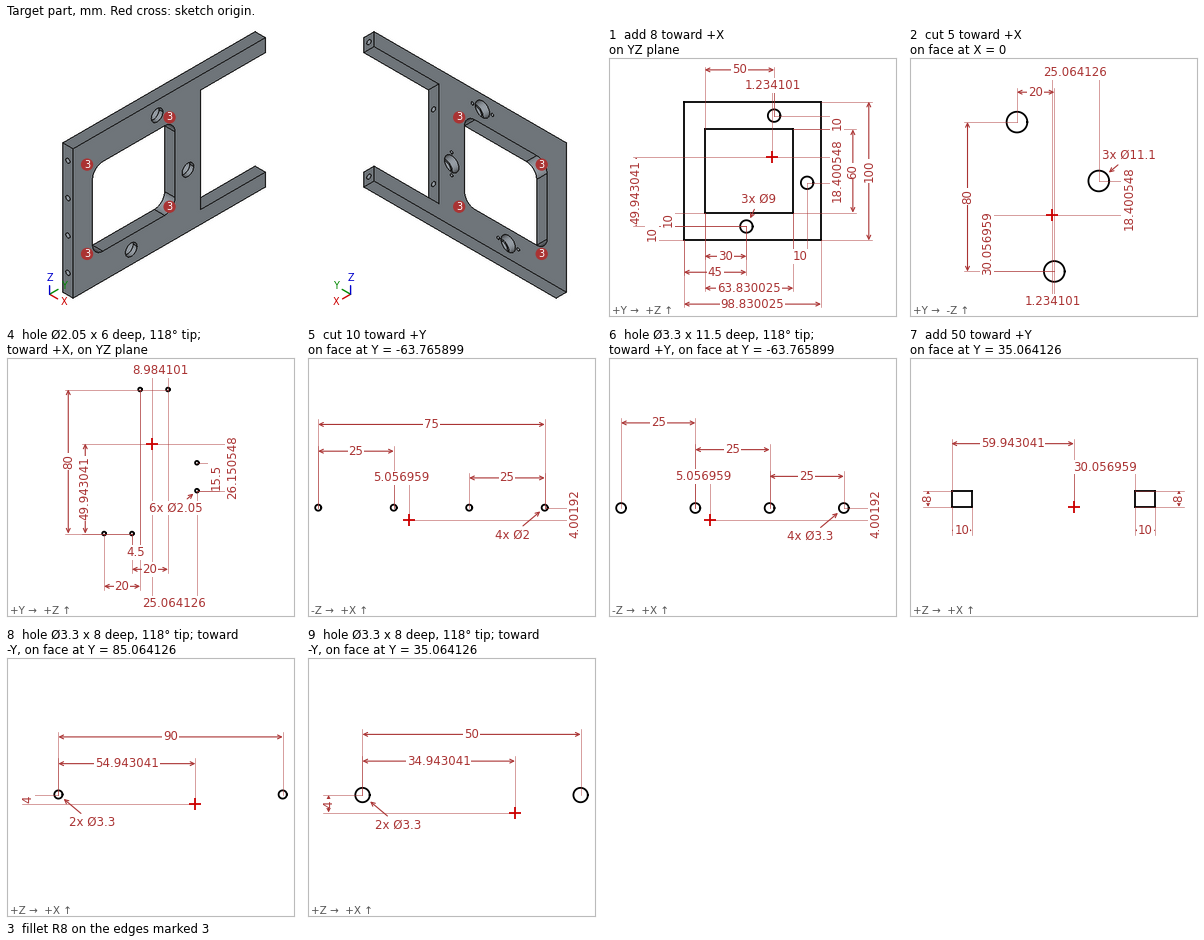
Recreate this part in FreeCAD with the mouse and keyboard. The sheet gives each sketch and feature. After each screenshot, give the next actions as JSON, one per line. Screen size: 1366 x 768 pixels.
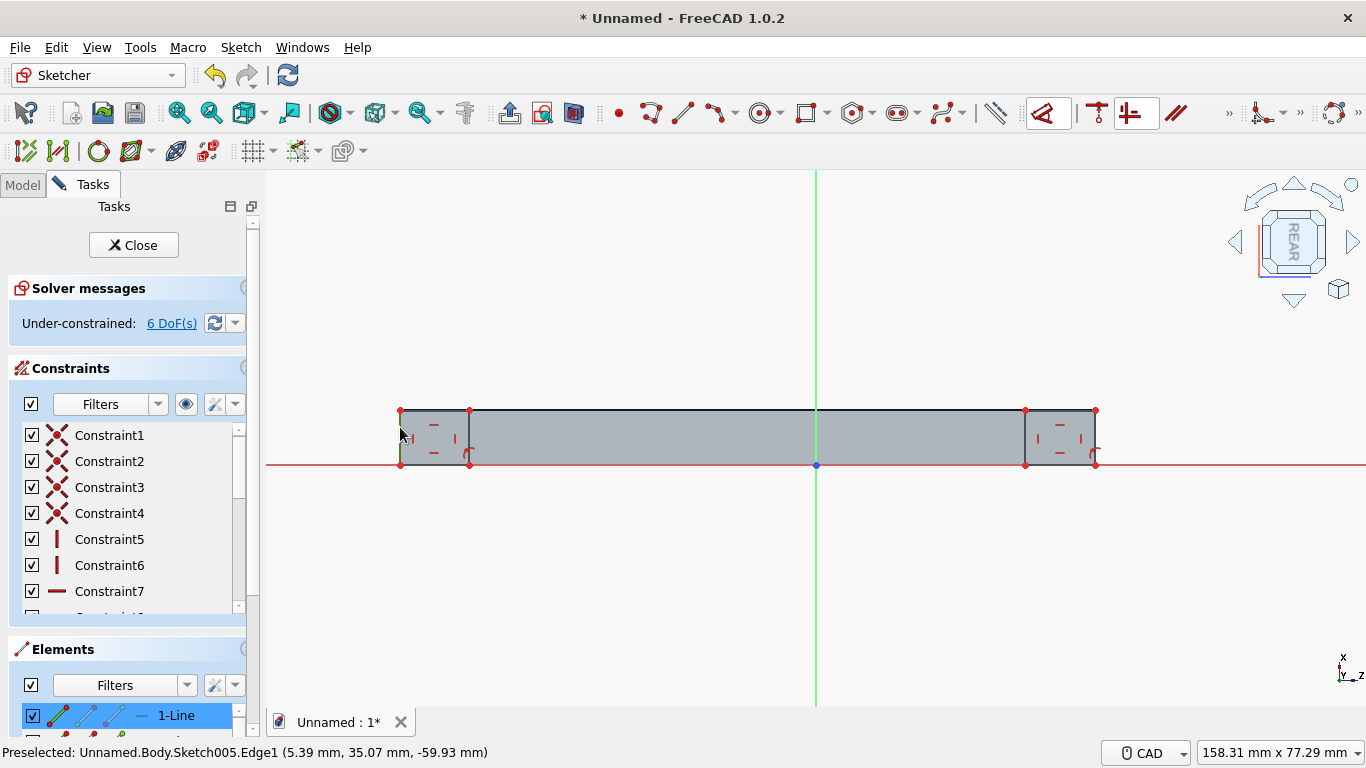
{"action": "left_click", "coordinate": [1066, 114]}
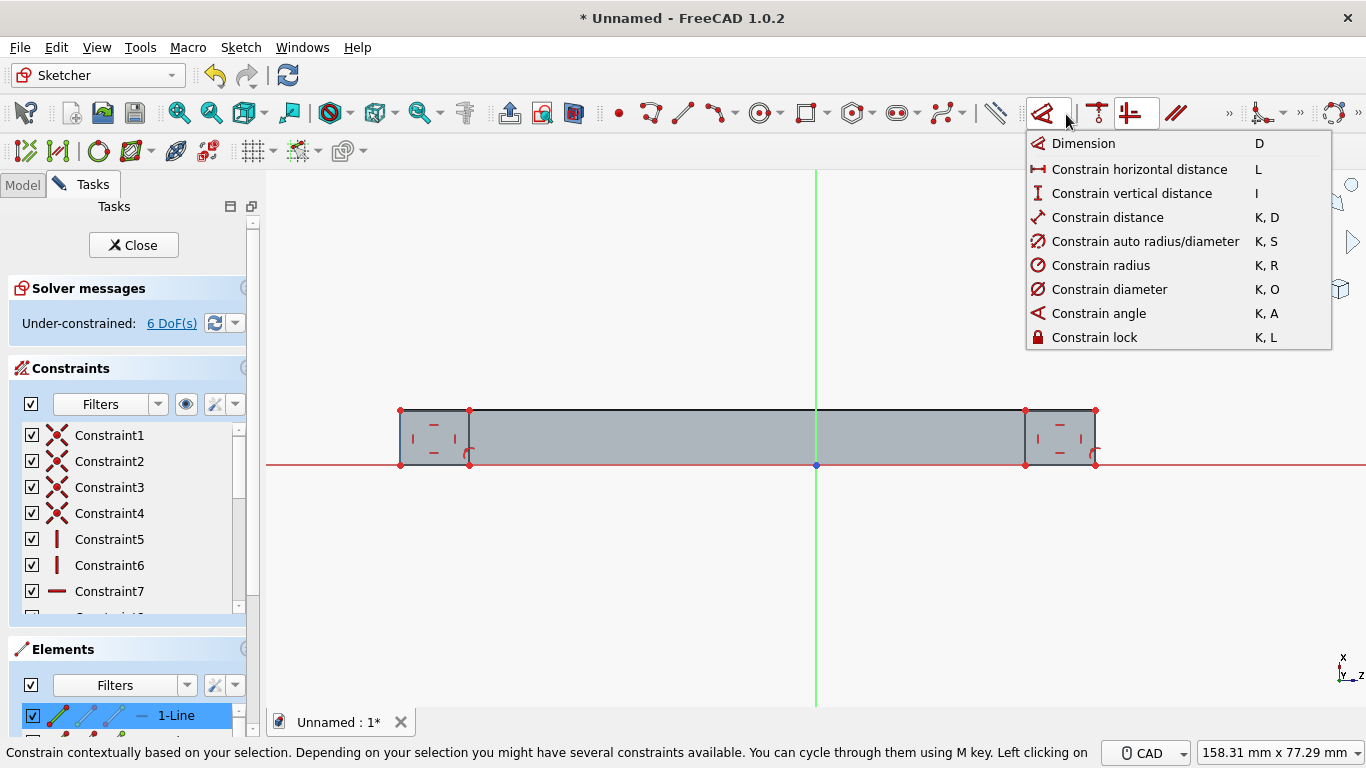
{"action": "left_click", "coordinate": [1179, 193]}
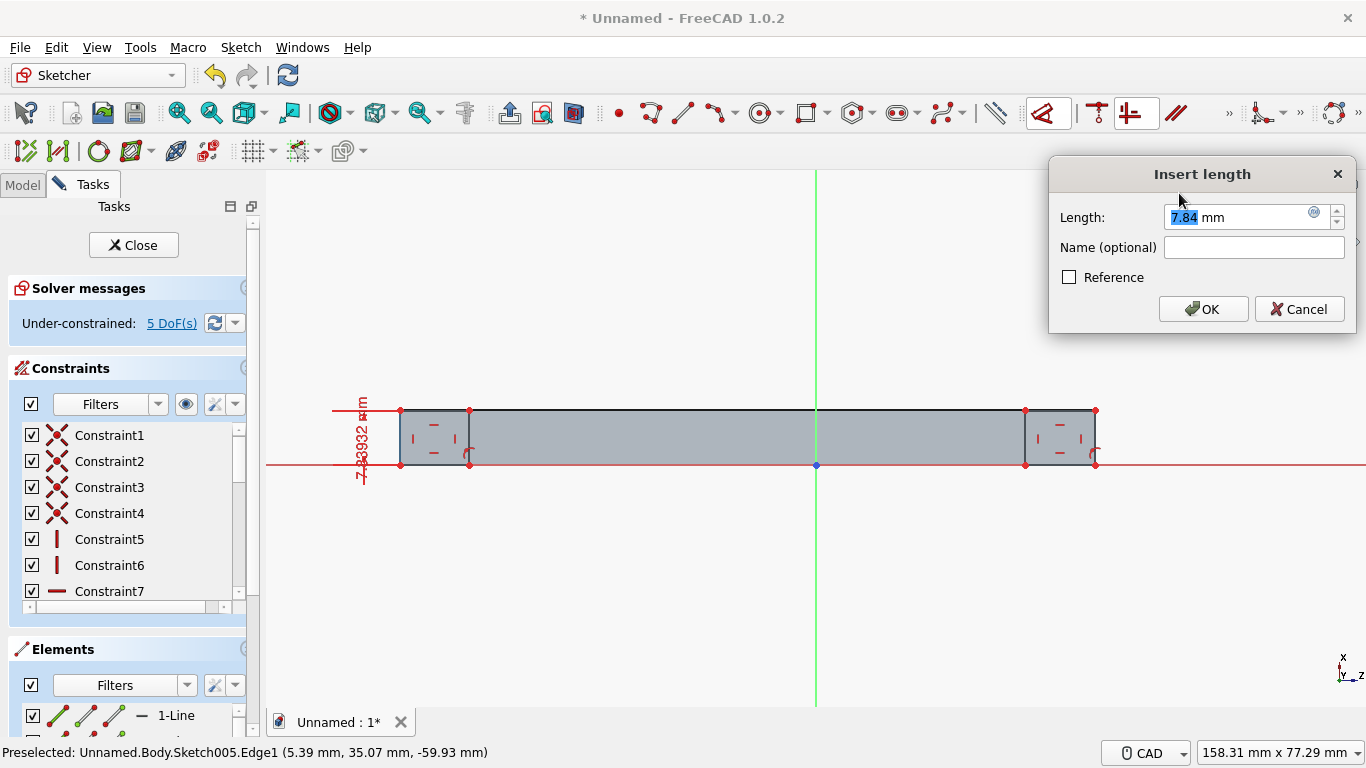
{"action": "type", "text": "8"}
{"action": "key", "text": "Return"}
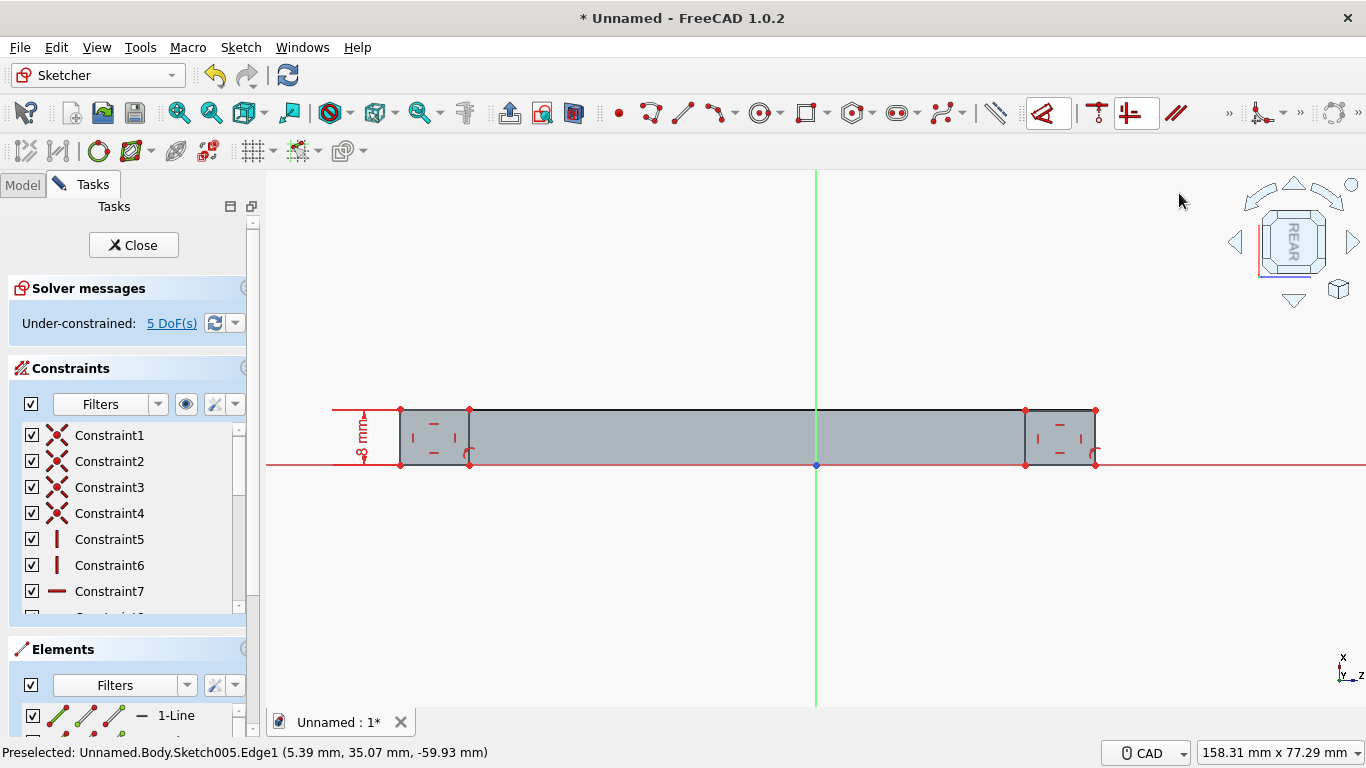
{"action": "left_click", "coordinate": [1025, 427]}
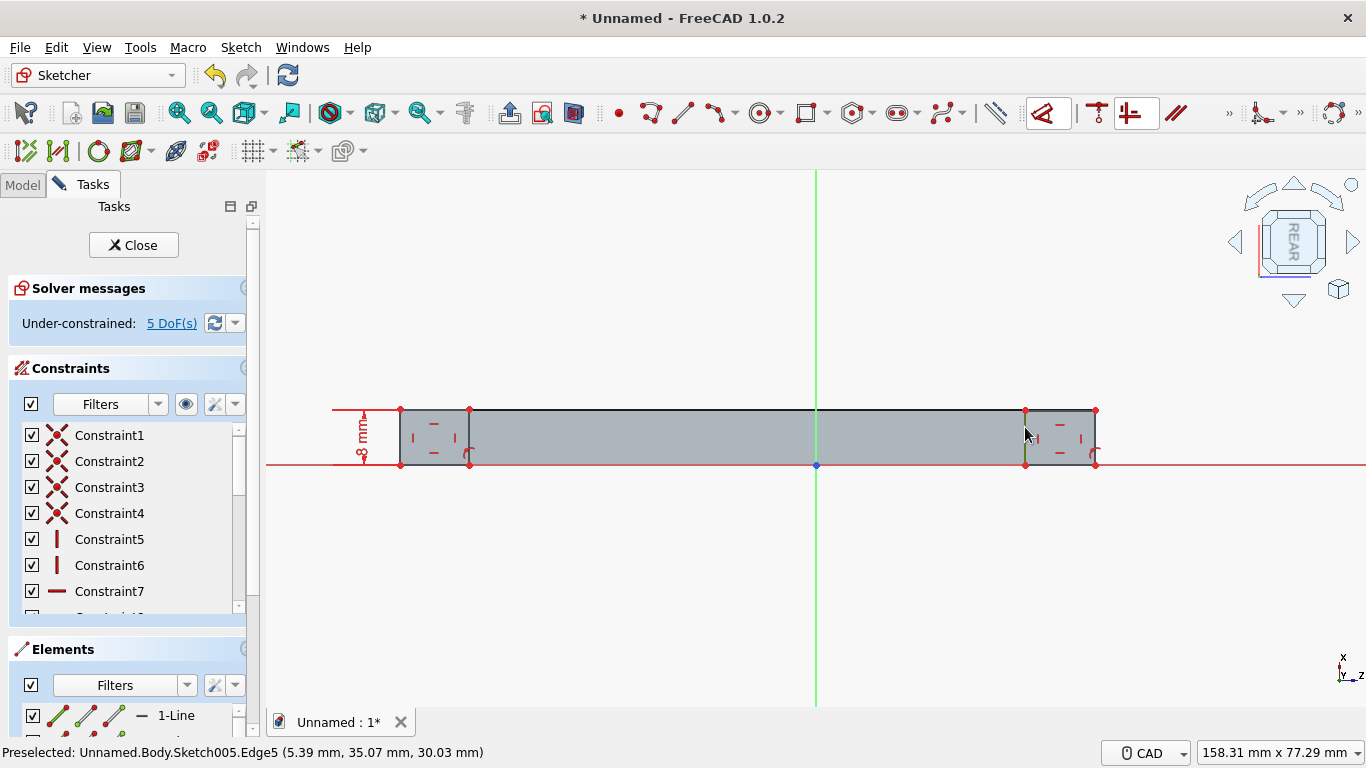
{"action": "key", "text": "i"}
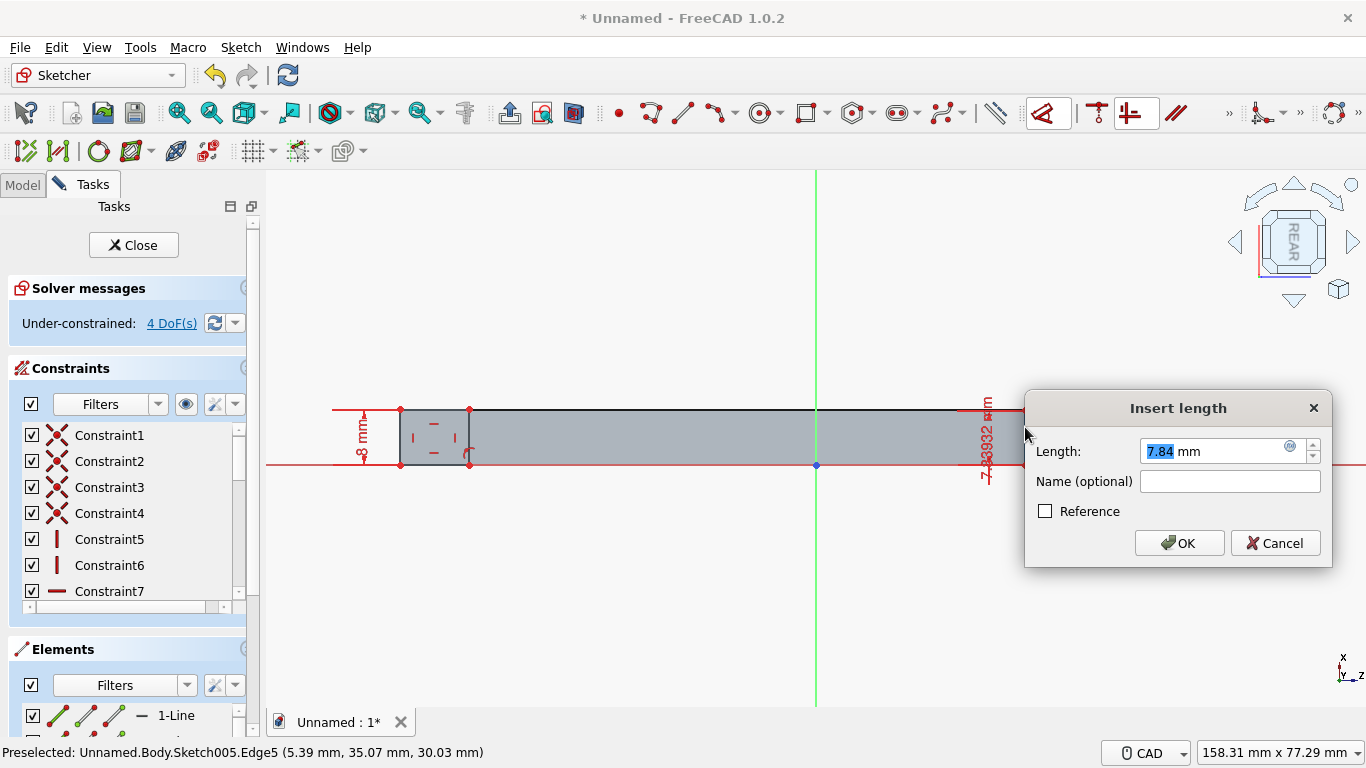
{"action": "type", "text": "8"}
{"action": "key", "text": "Return"}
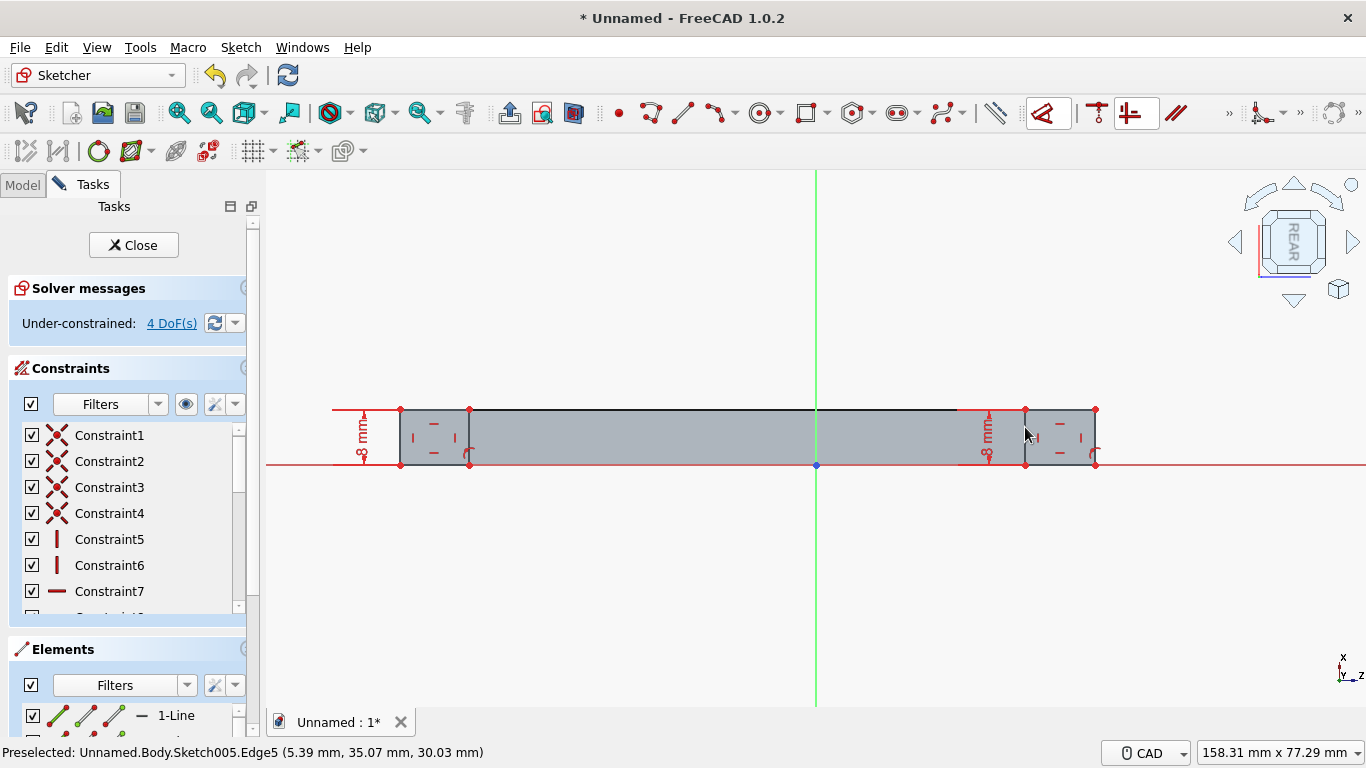
{"action": "left_click", "coordinate": [421, 465]}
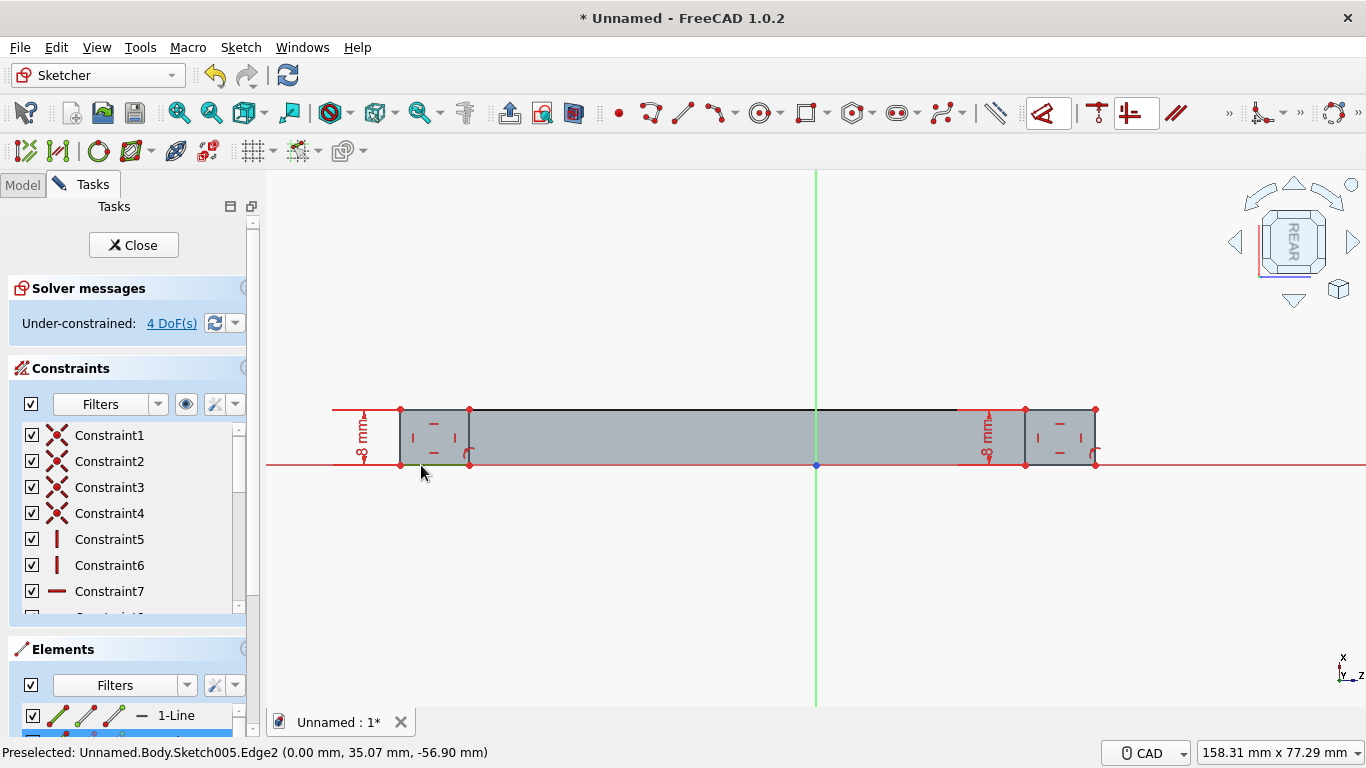
{"action": "left_click", "coordinate": [1066, 114]}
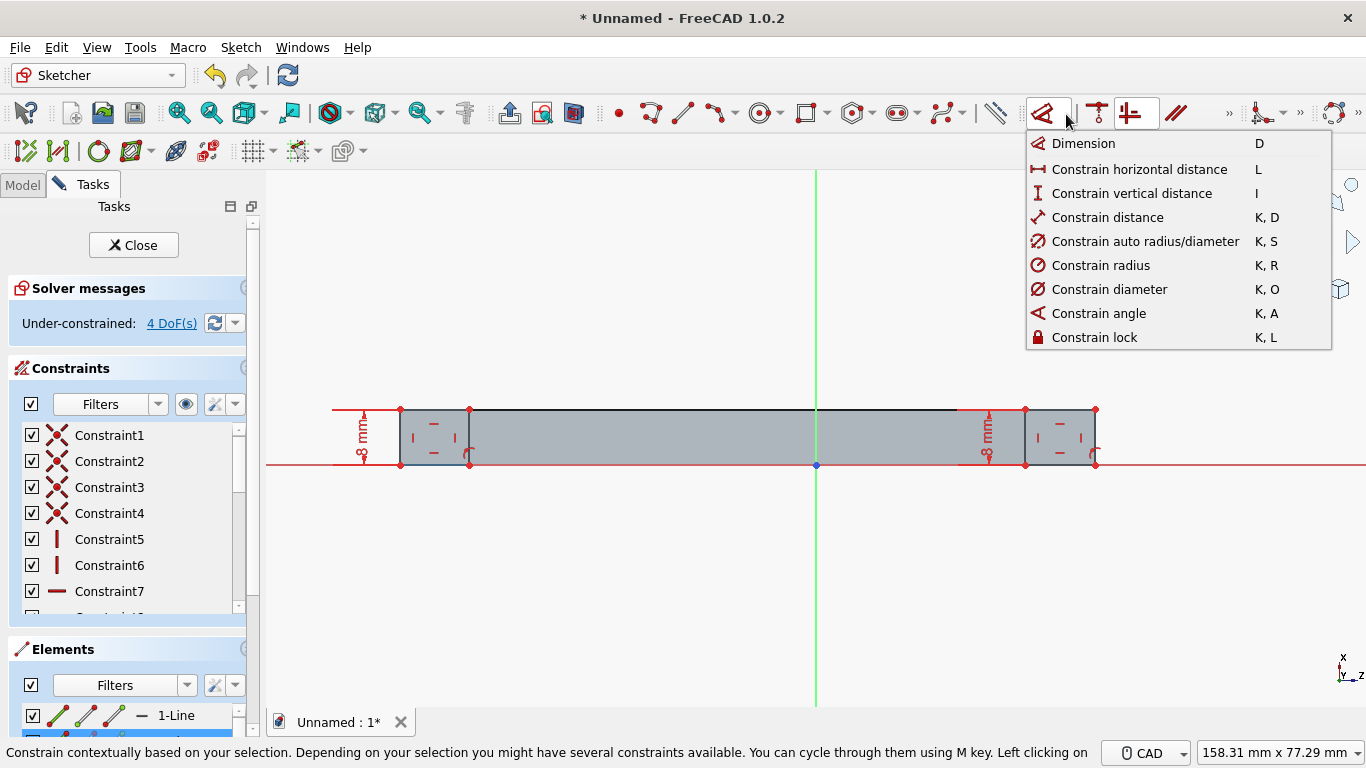
{"action": "left_click", "coordinate": [1179, 169]}